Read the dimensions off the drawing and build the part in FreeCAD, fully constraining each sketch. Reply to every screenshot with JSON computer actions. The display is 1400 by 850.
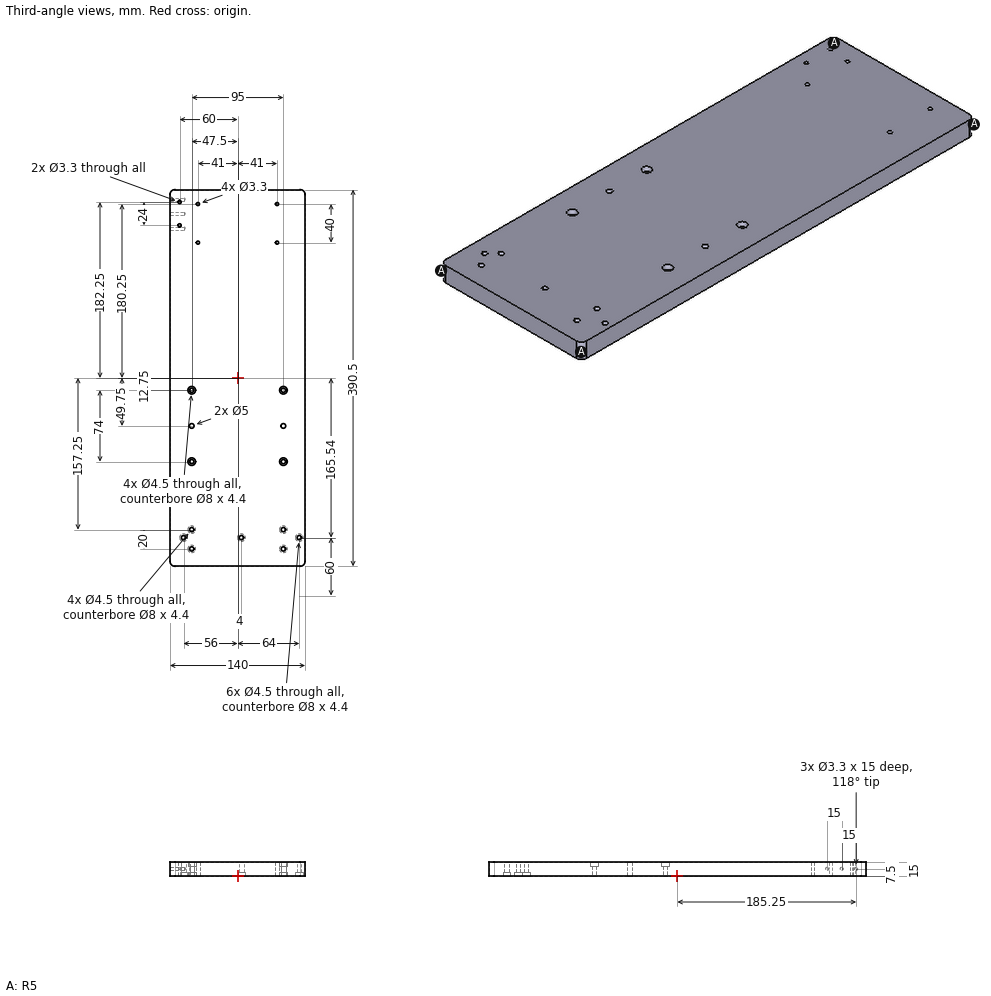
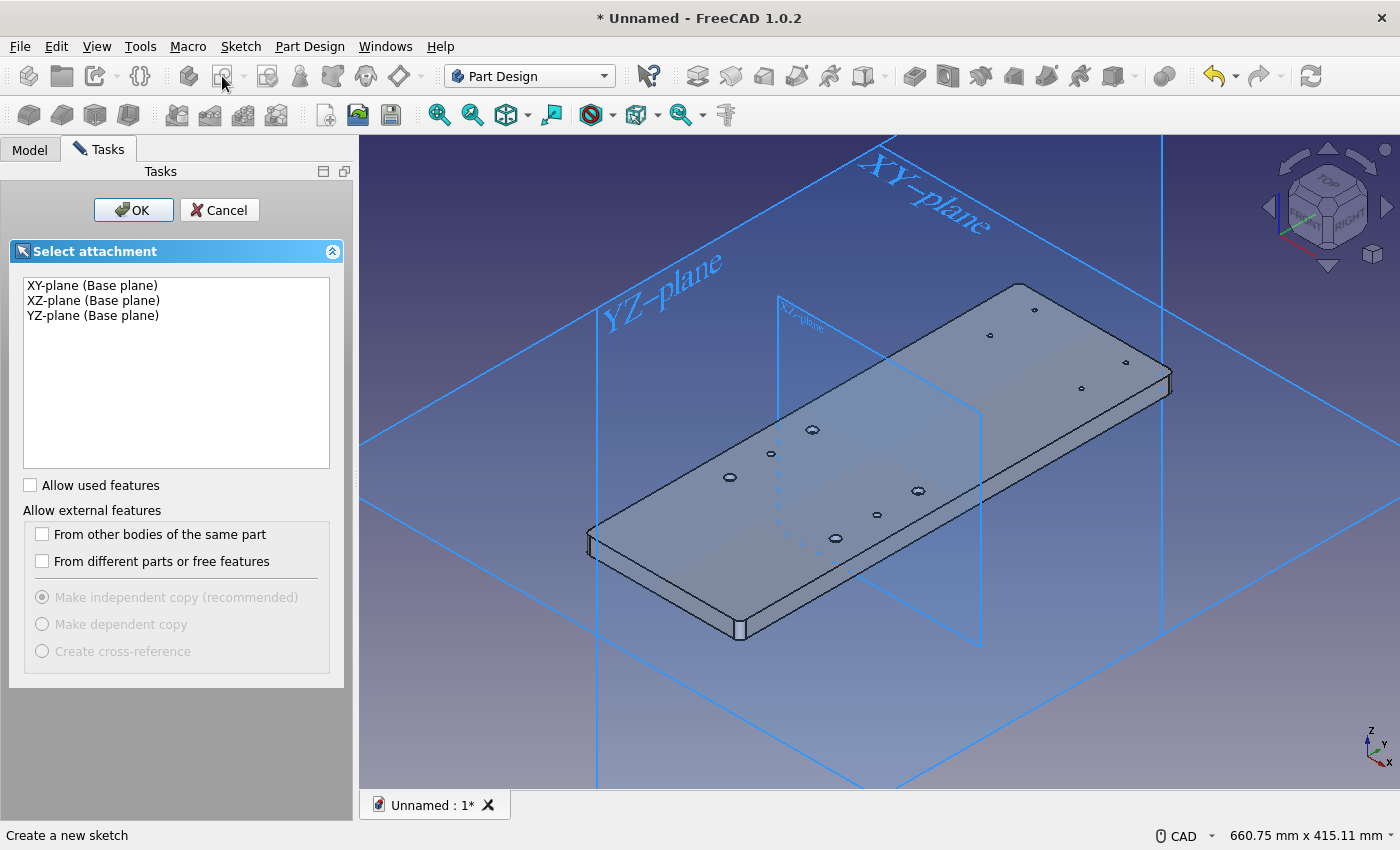
{"action": "left_click", "coordinate": [84, 286]}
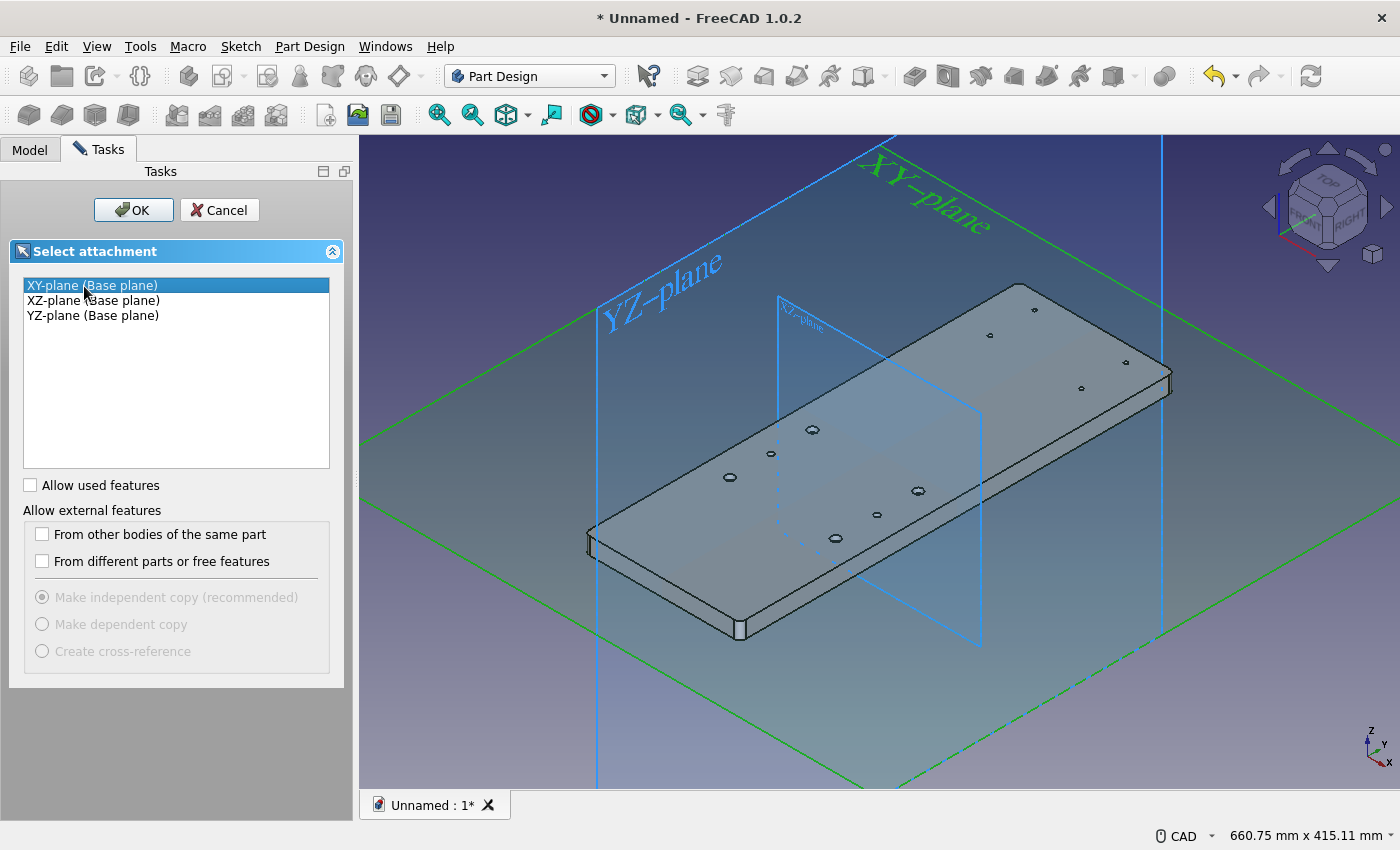
{"action": "left_click", "coordinate": [134, 210]}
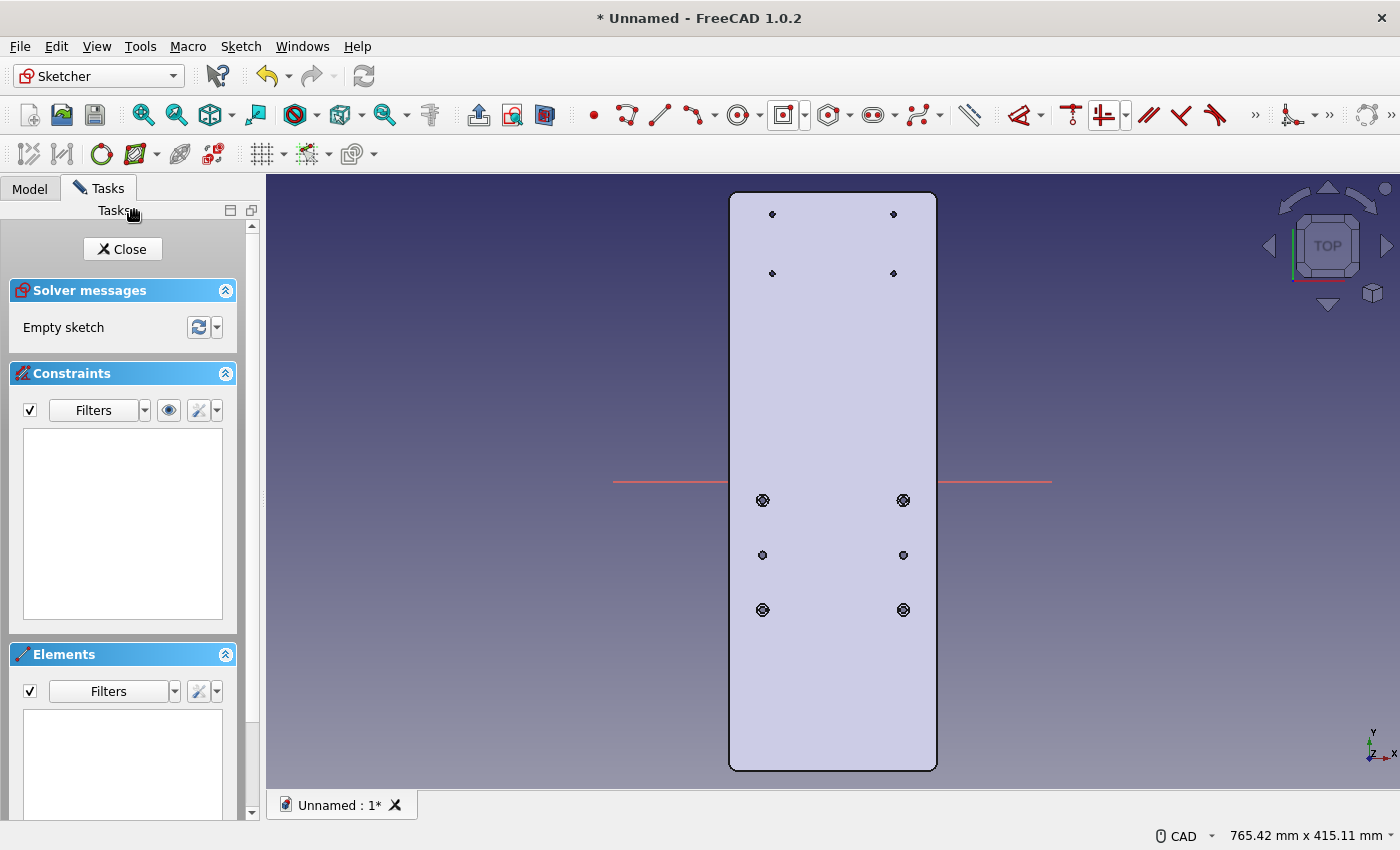
{"action": "left_click", "coordinate": [545, 116]}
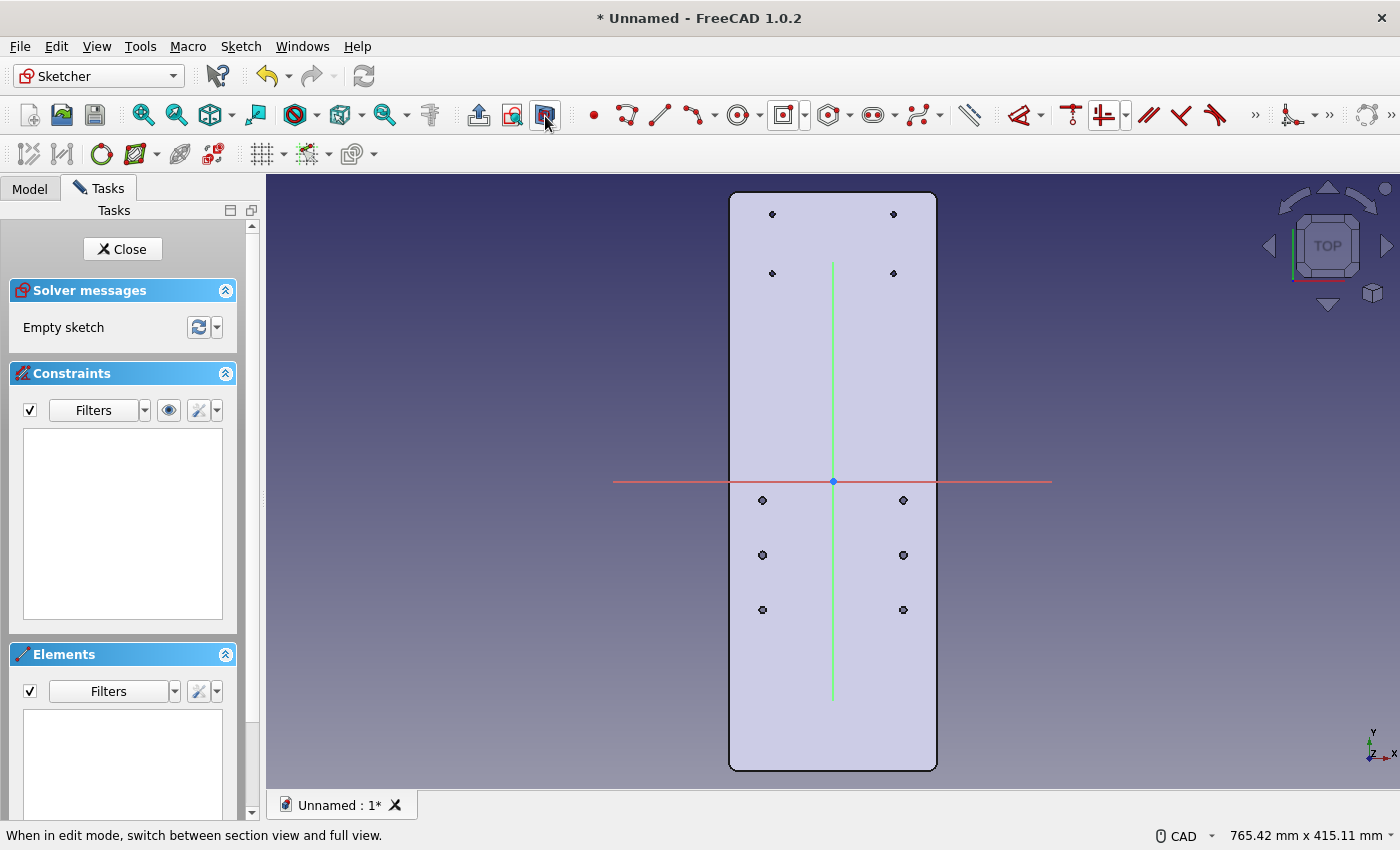
{"action": "scroll", "coordinate": [455, 202], "scroll_direction": "down", "scroll_amount": 1}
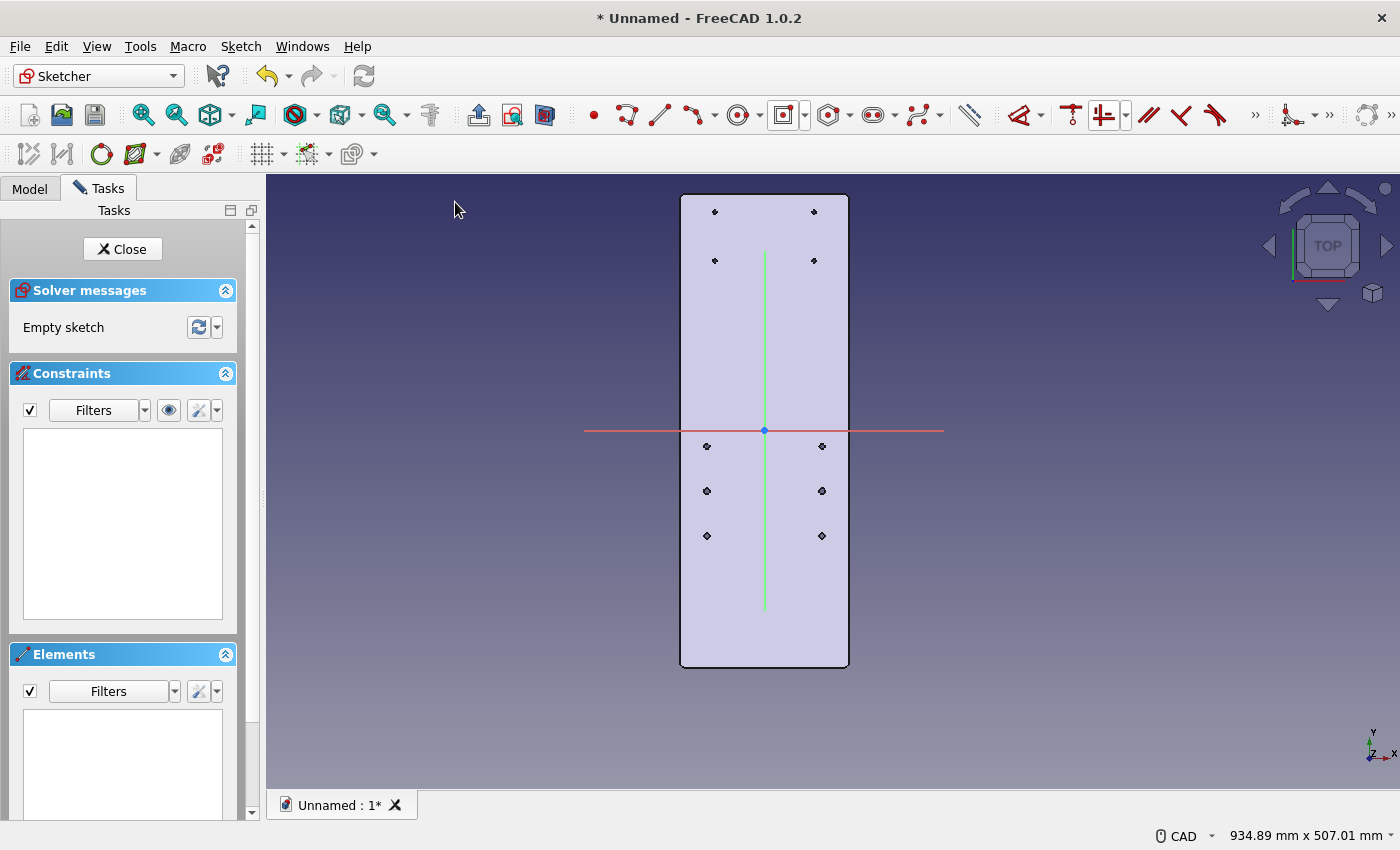
{"action": "scroll", "coordinate": [765, 611], "scroll_direction": "up", "scroll_amount": 3}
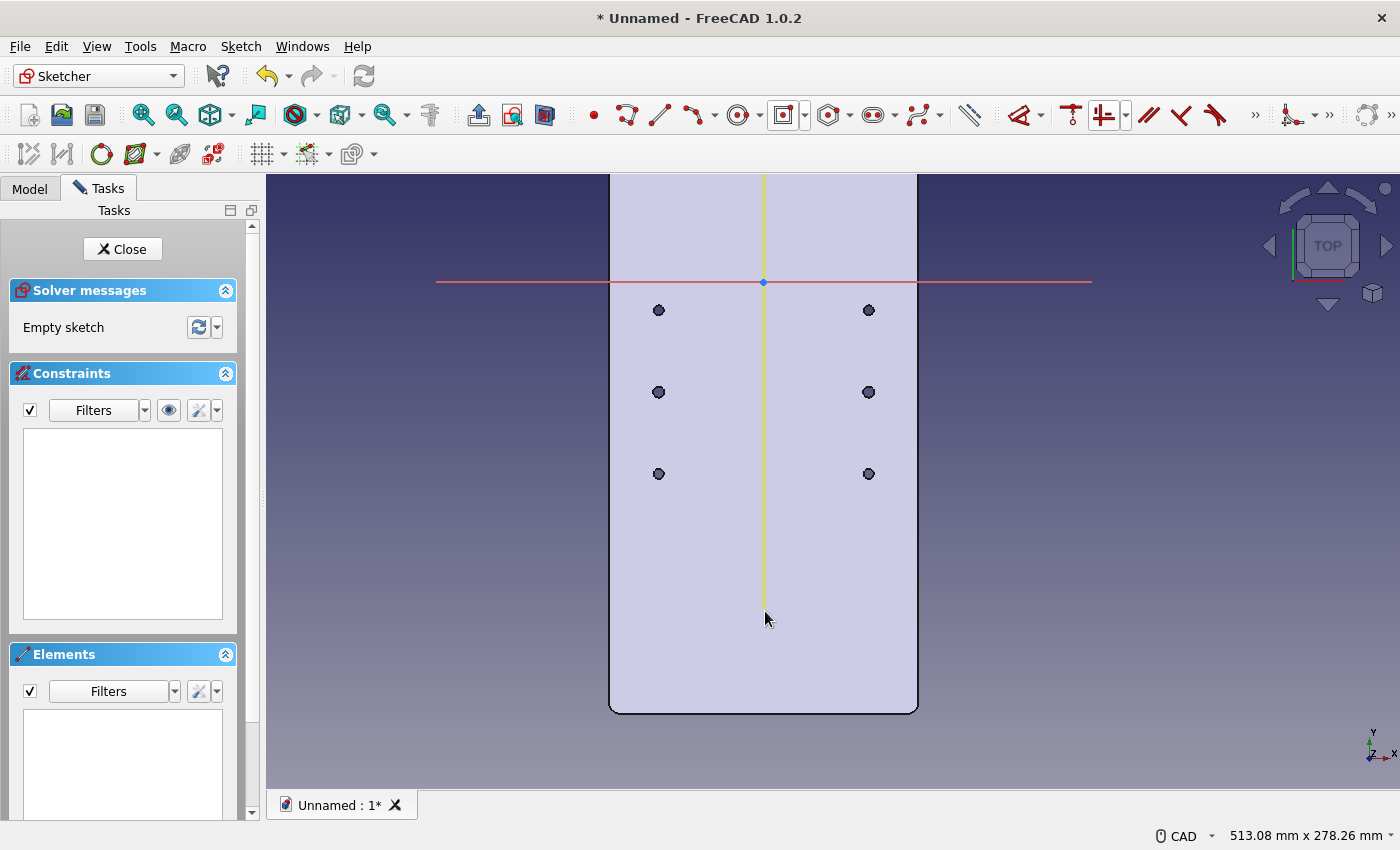
{"action": "left_click", "coordinate": [738, 116]}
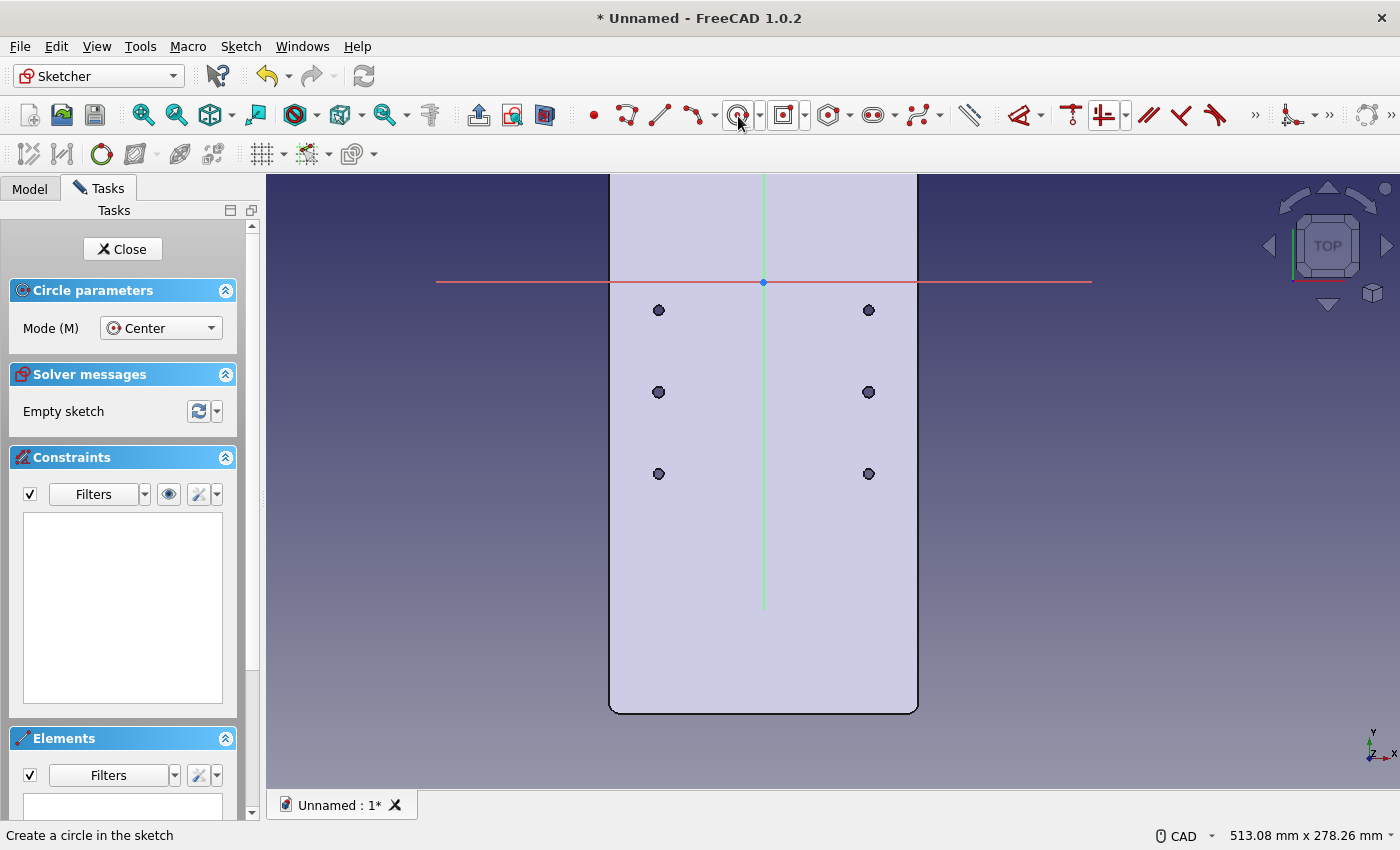
{"action": "scroll", "coordinate": [659, 630], "scroll_direction": "up", "scroll_amount": 8}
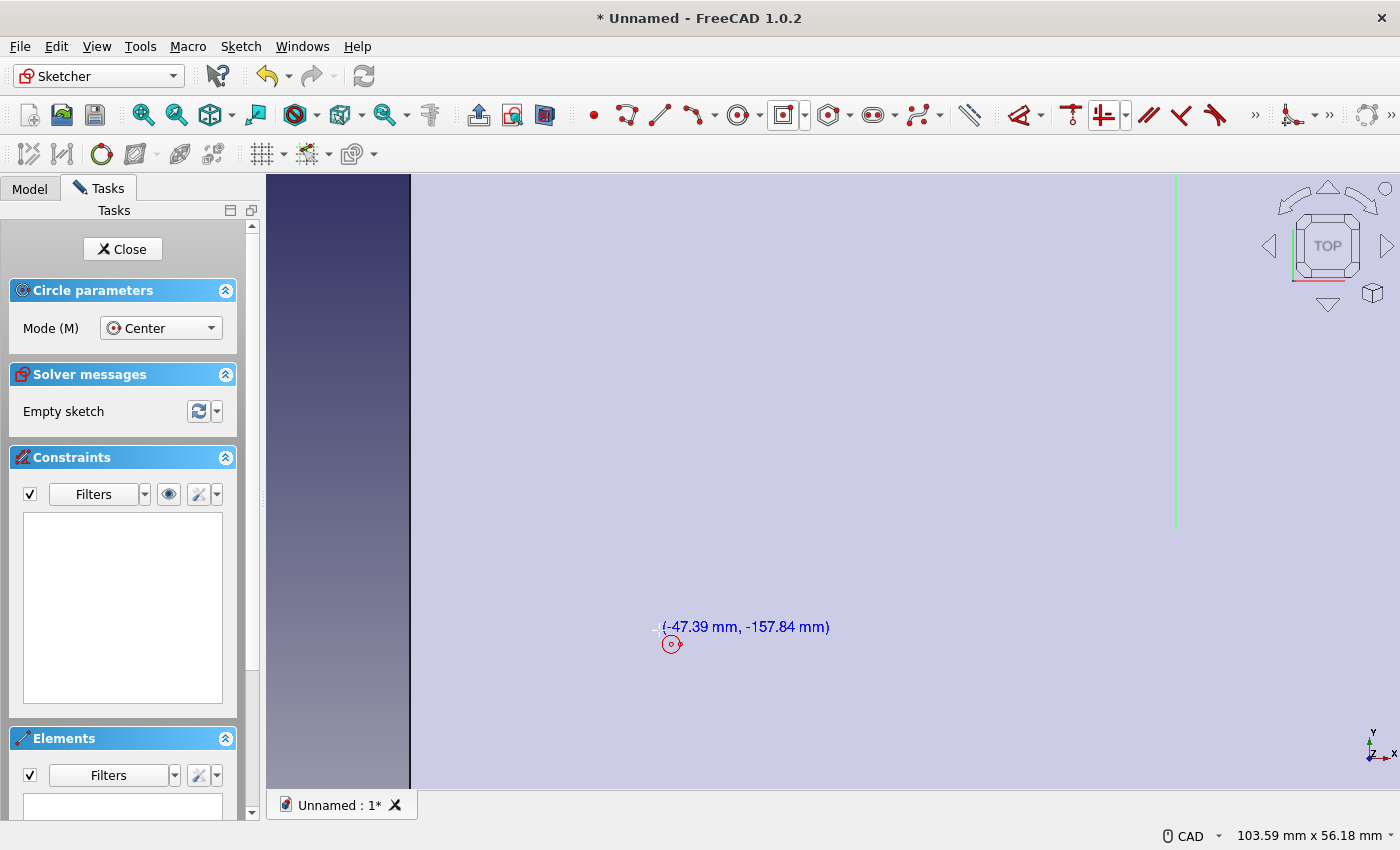
{"action": "scroll", "coordinate": [660, 632], "scroll_direction": "down", "scroll_amount": 8}